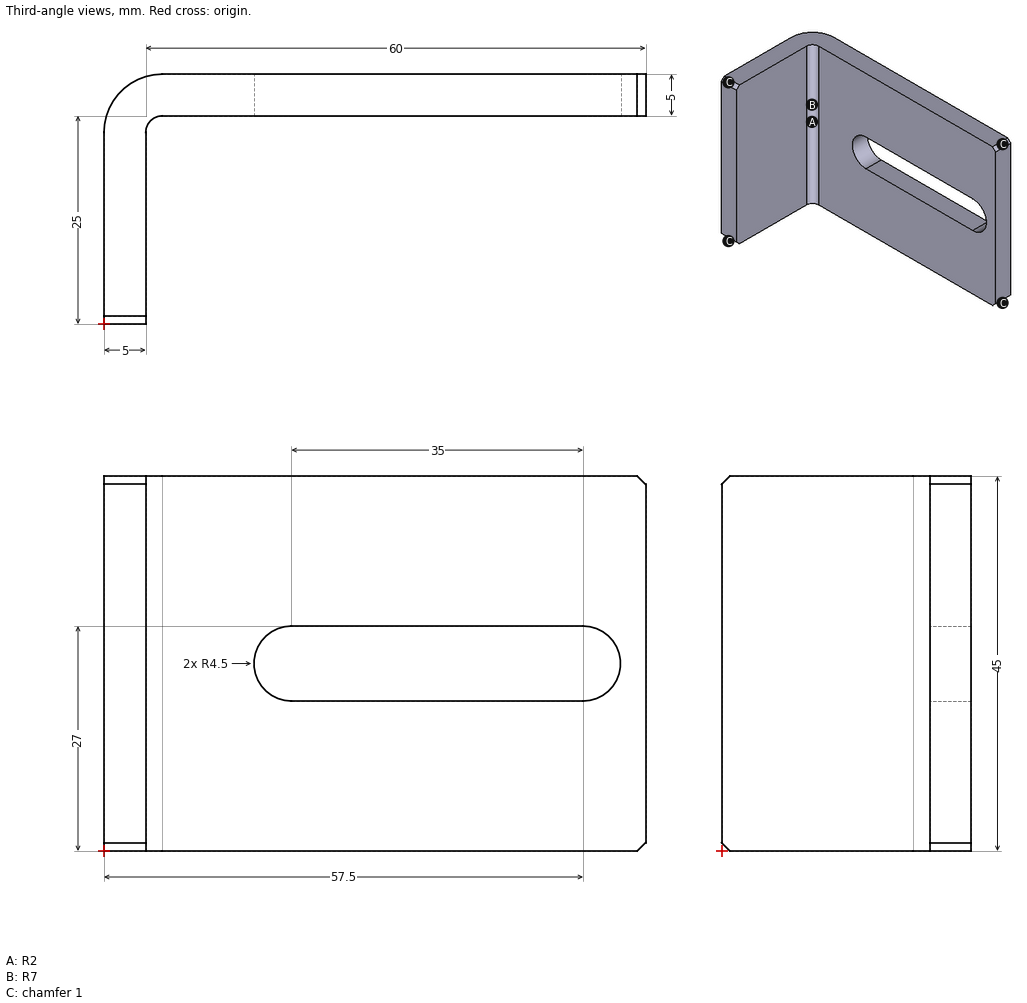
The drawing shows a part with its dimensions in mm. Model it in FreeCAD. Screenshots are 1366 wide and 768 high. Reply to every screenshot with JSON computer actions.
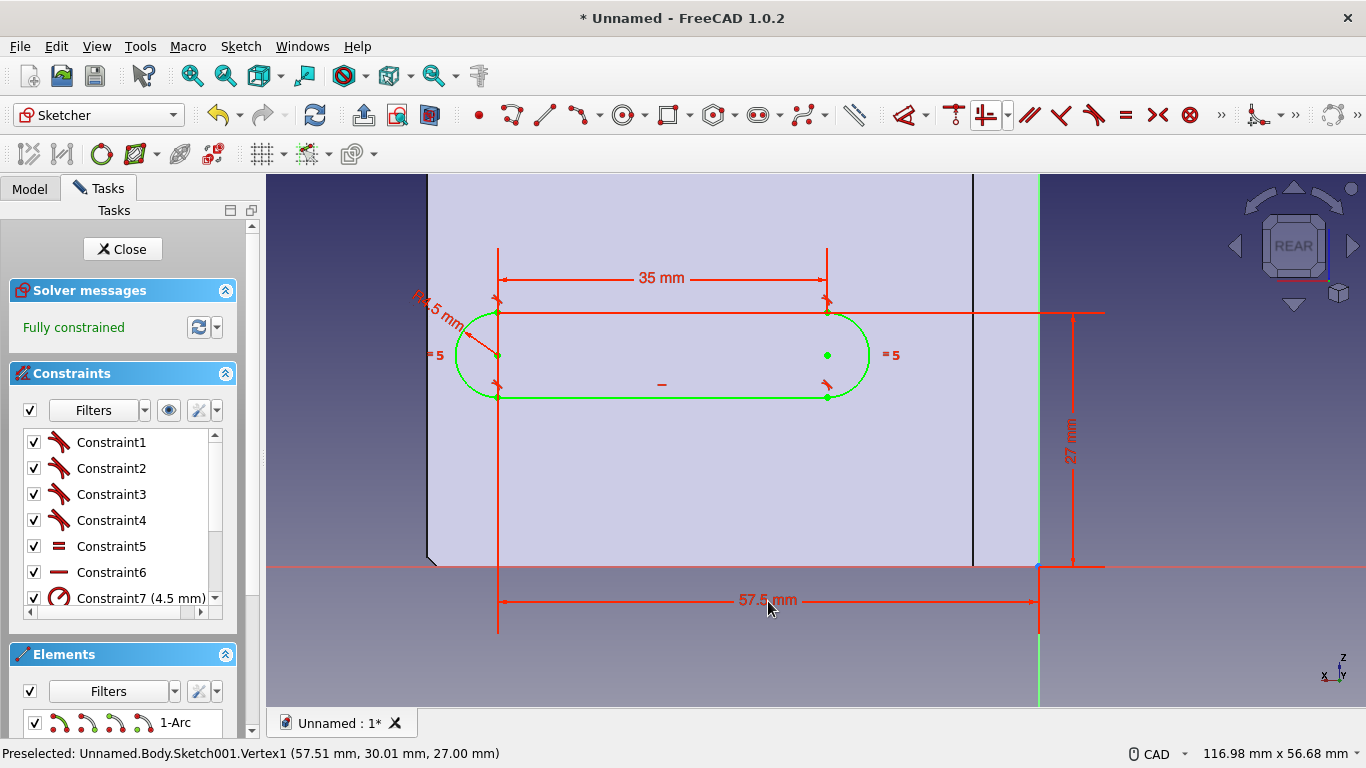
{"action": "left_click", "coordinate": [123, 249]}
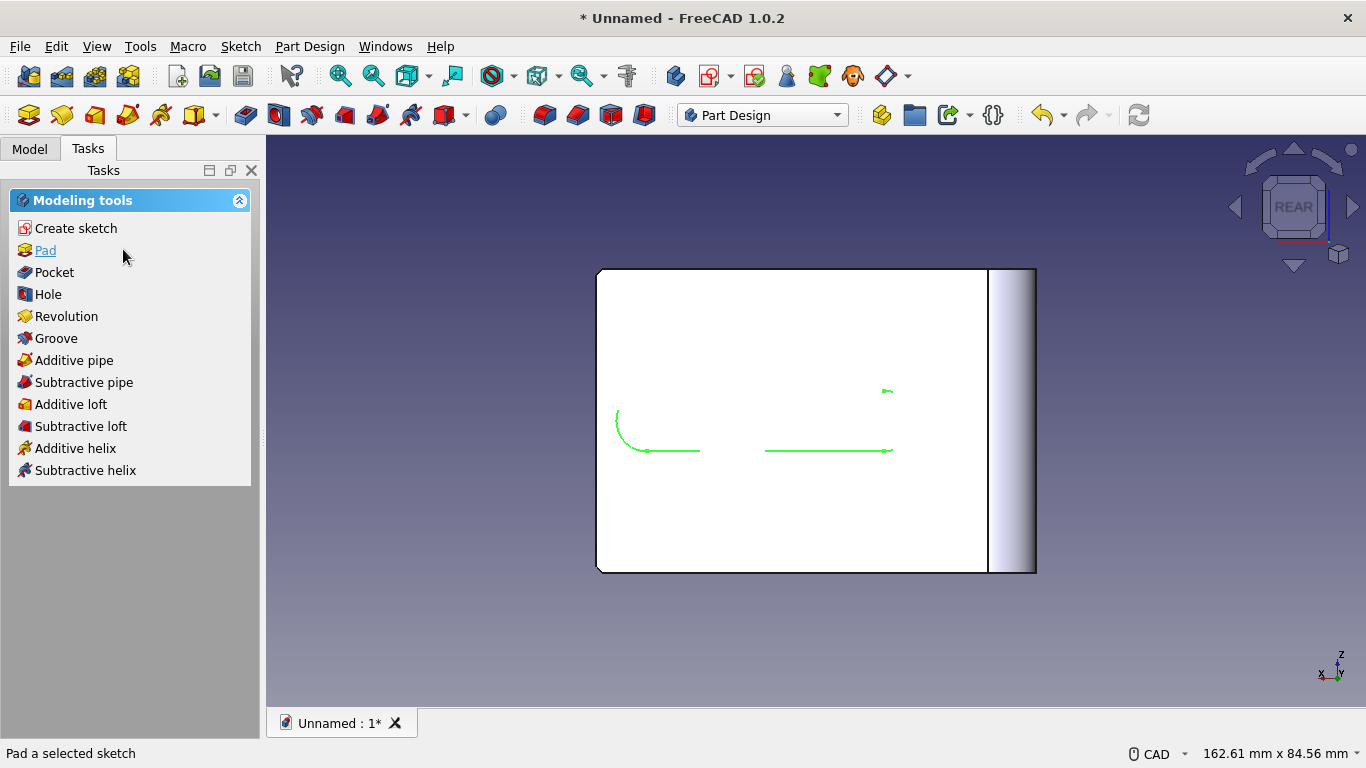
{"action": "left_click", "coordinate": [246, 116]}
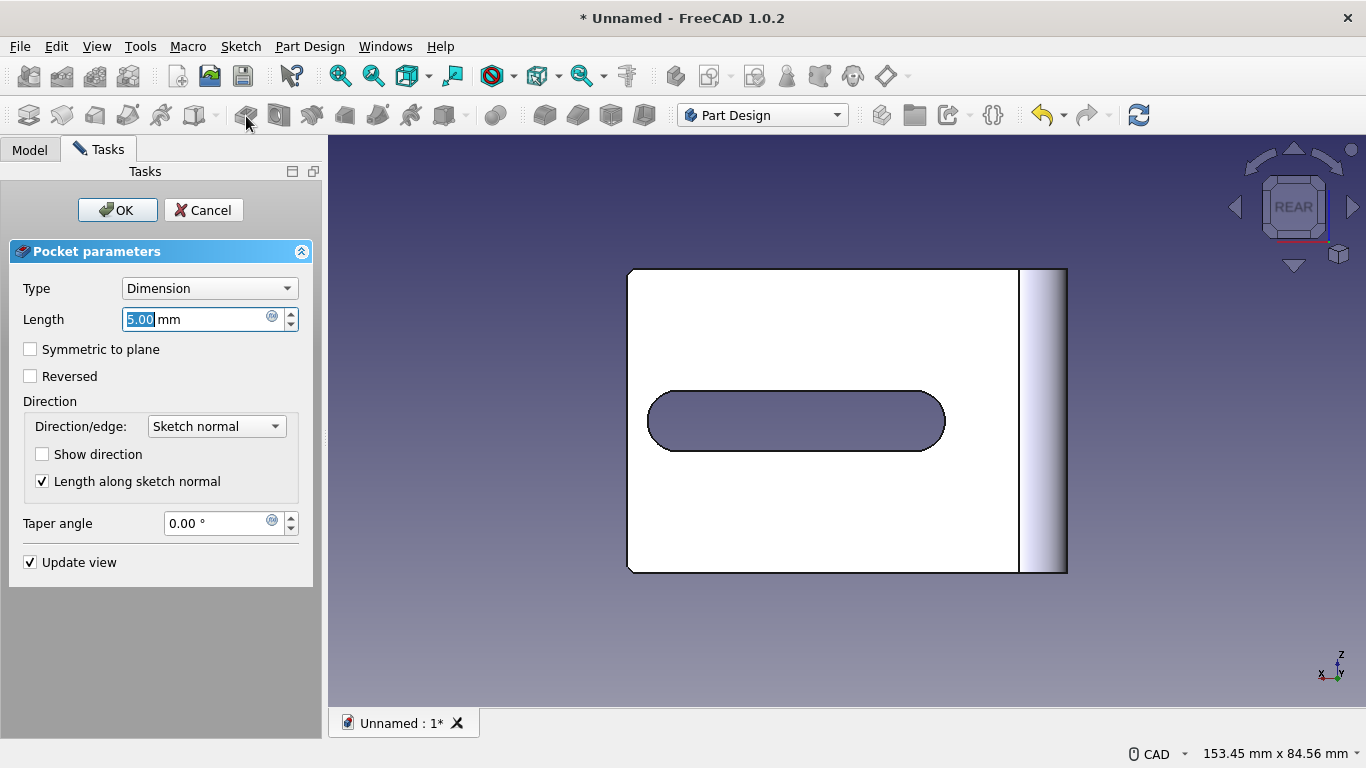
{"action": "left_click", "coordinate": [210, 288]}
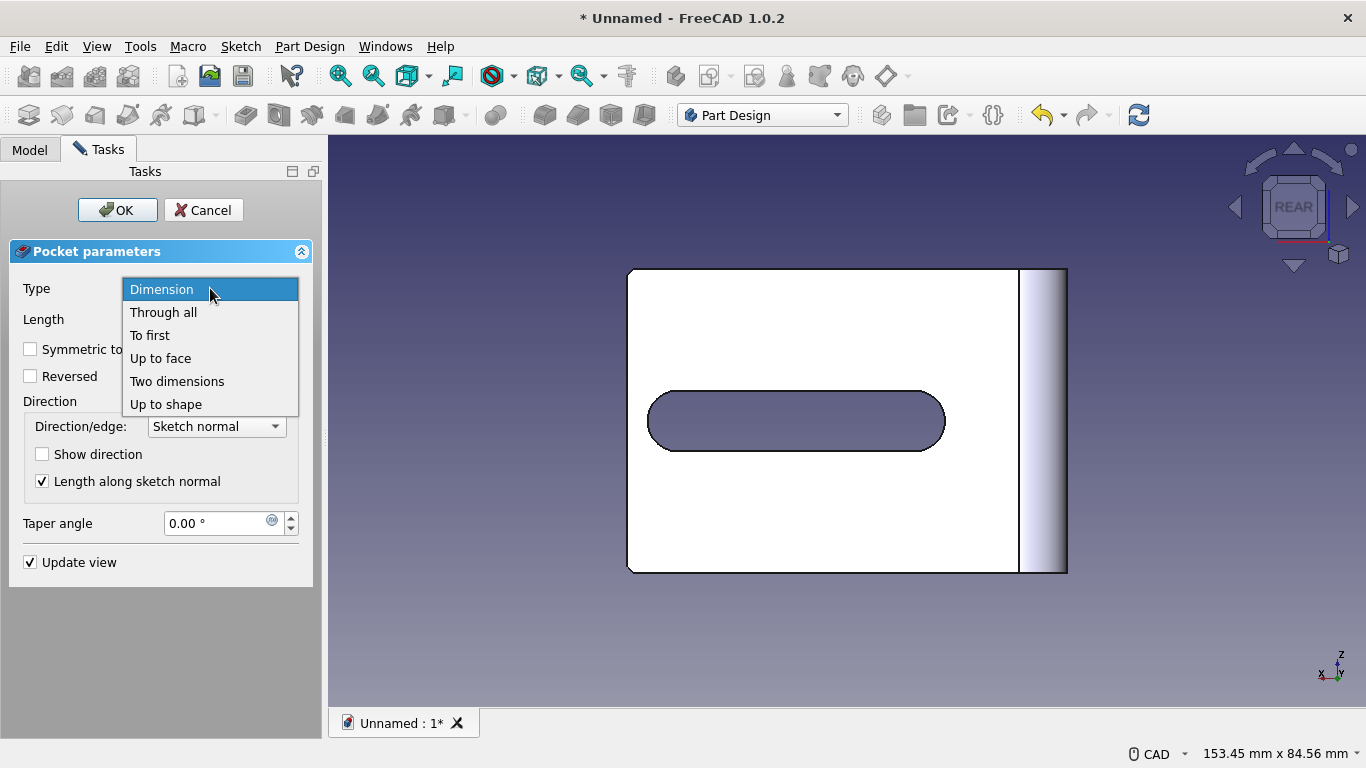
{"action": "left_click", "coordinate": [208, 312]}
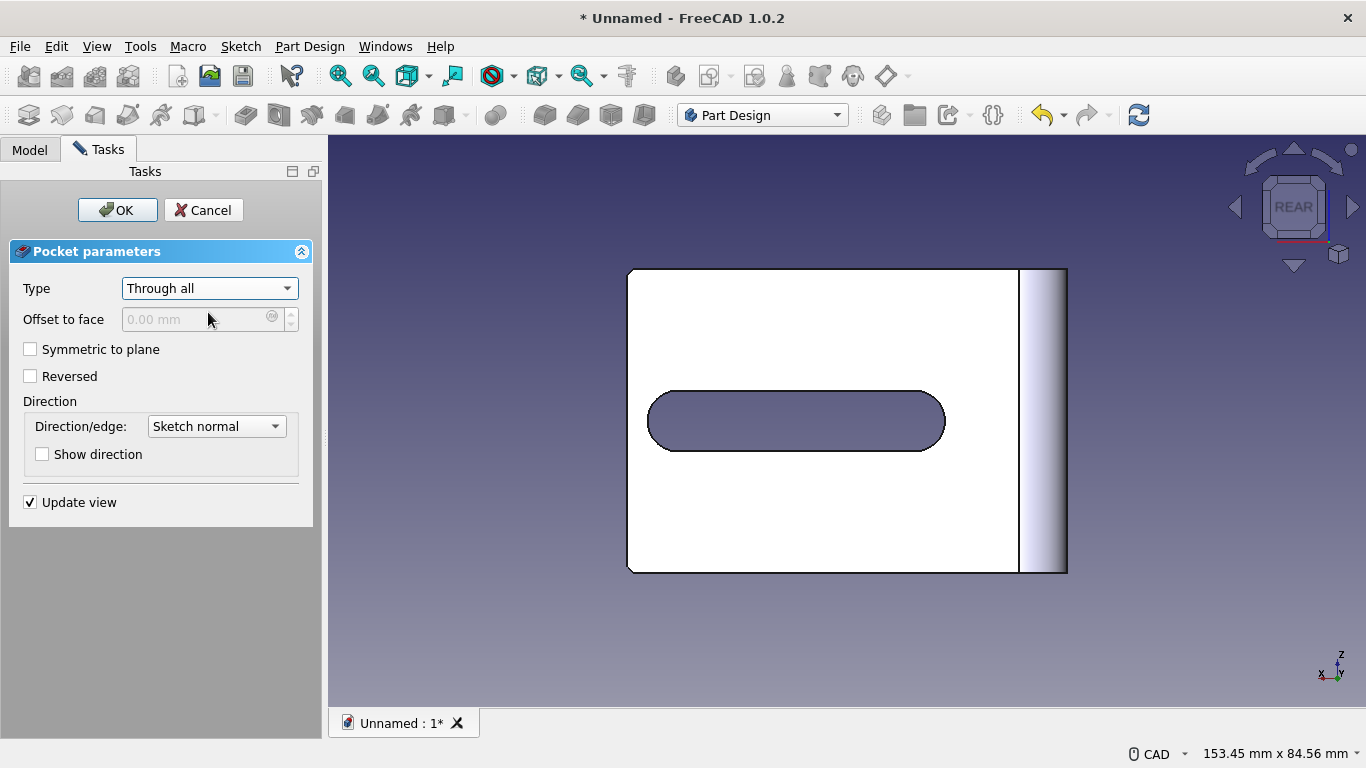
{"action": "left_click", "coordinate": [118, 210]}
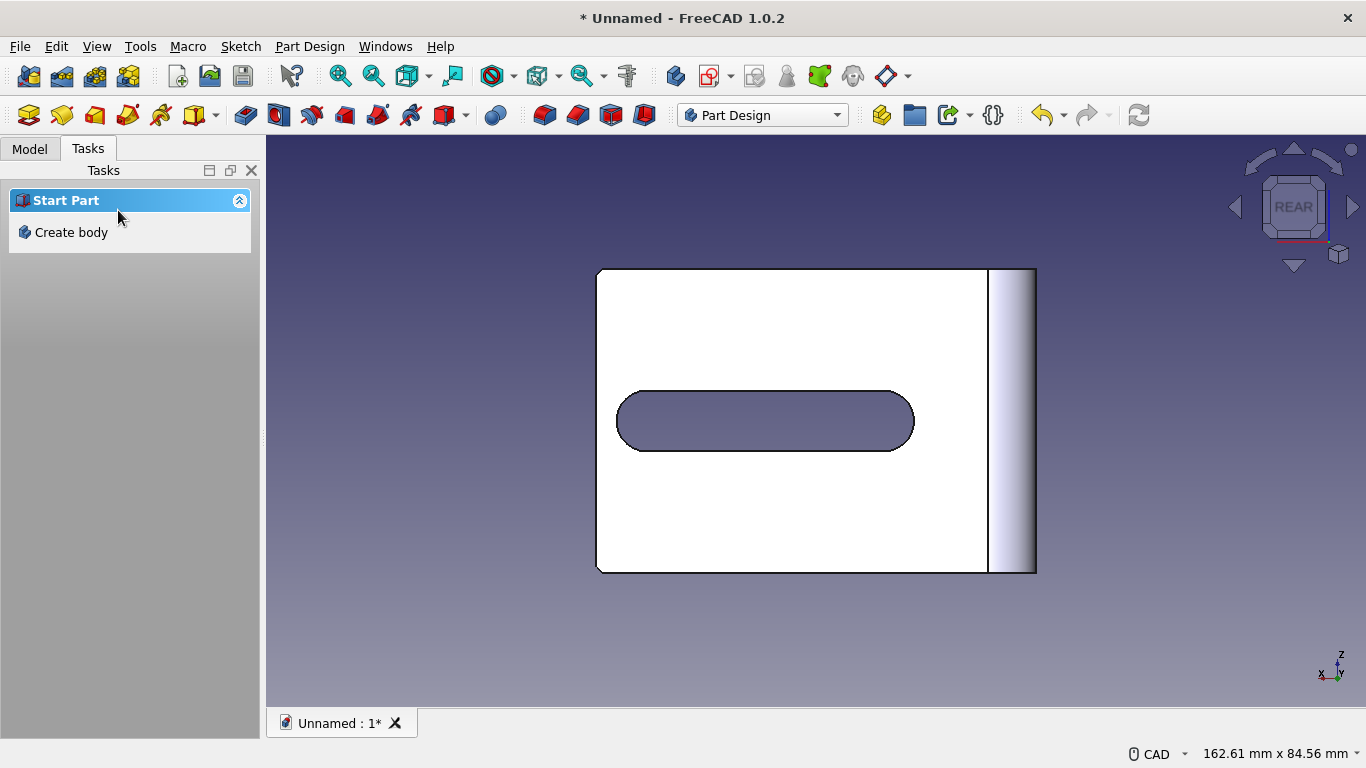
{"action": "key", "text": "0"}